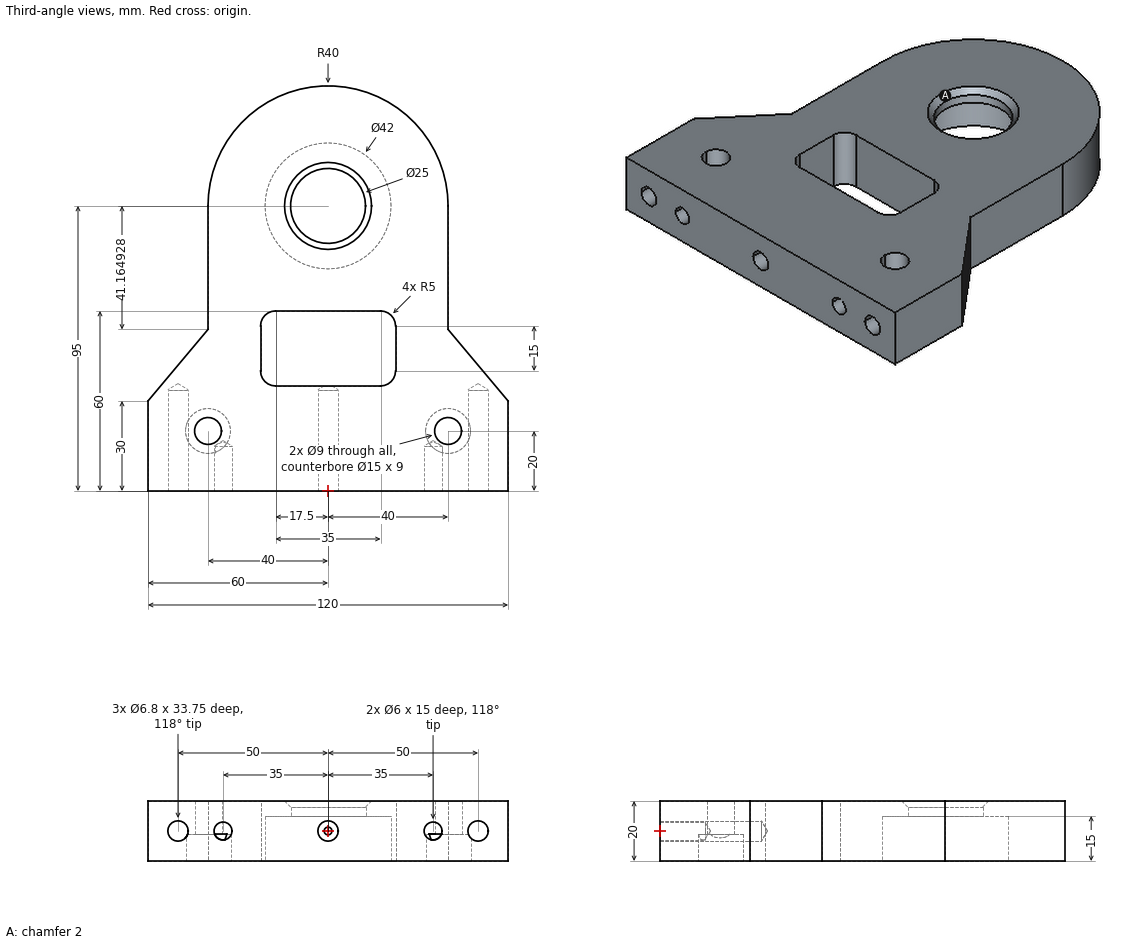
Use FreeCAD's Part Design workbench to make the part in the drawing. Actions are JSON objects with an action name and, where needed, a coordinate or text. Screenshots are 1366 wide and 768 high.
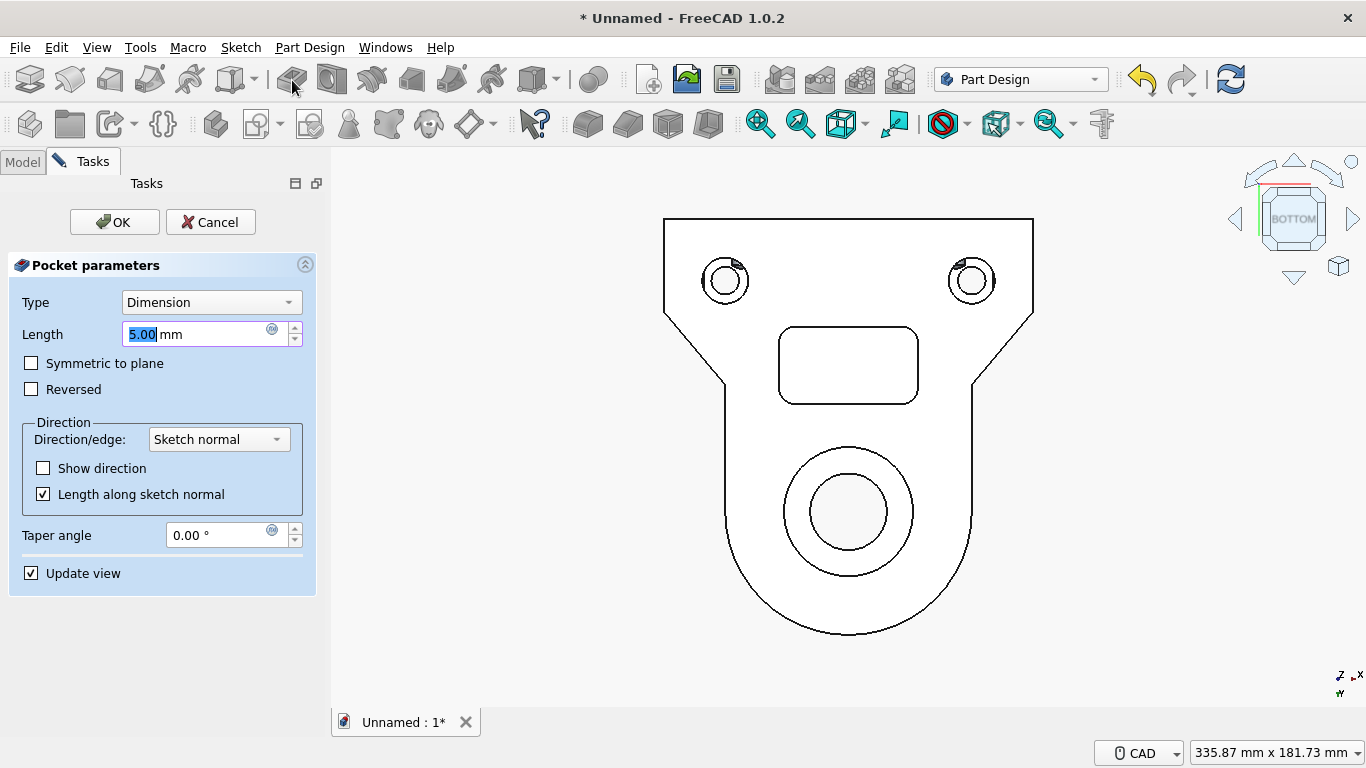
{"action": "left_click", "coordinate": [212, 302]}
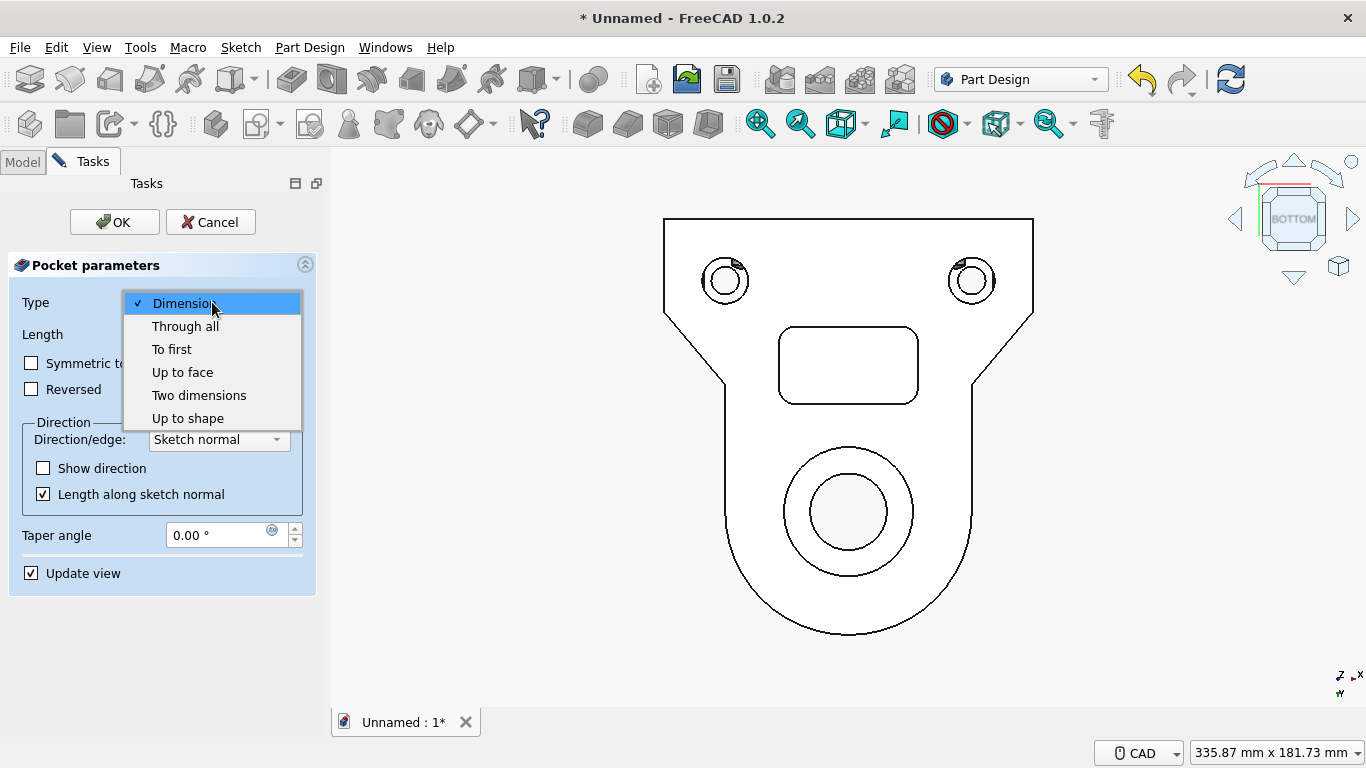
{"action": "left_click", "coordinate": [212, 326]}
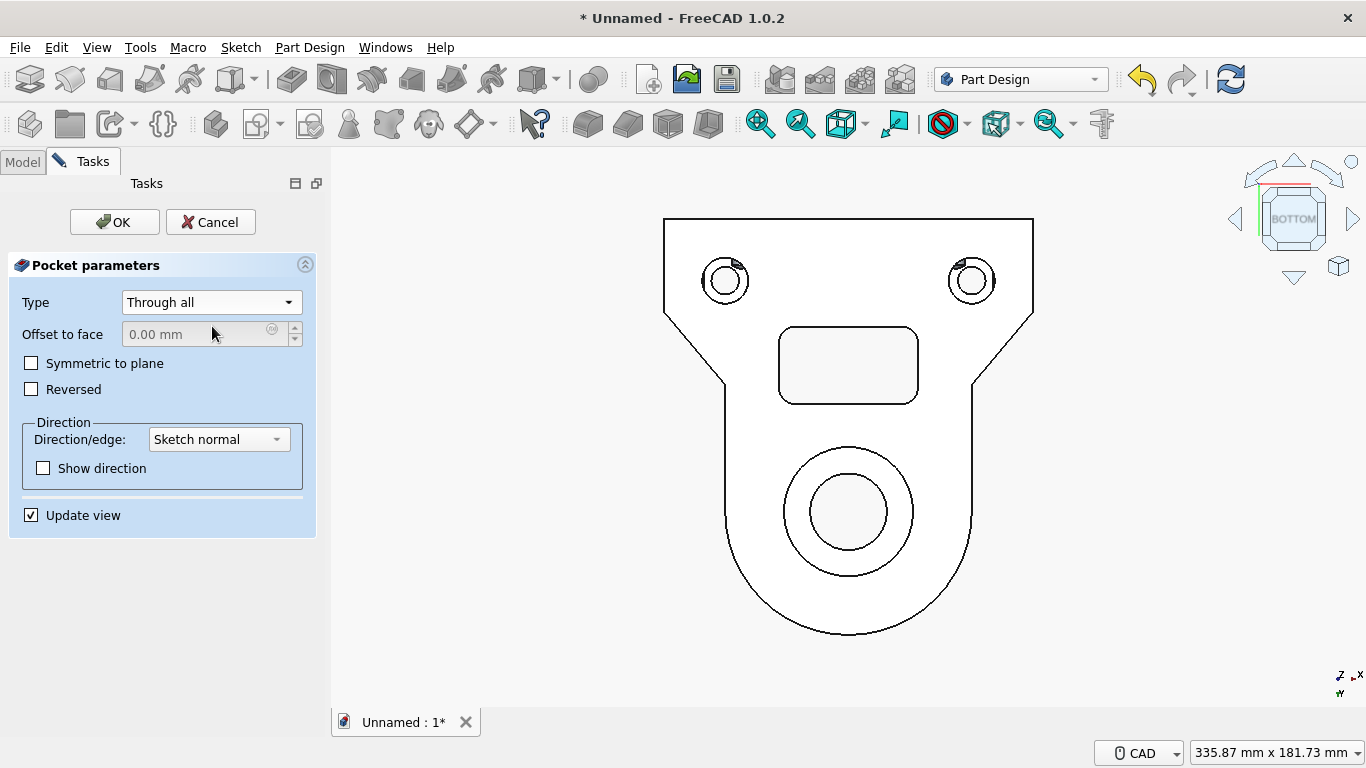
{"action": "left_click", "coordinate": [115, 222]}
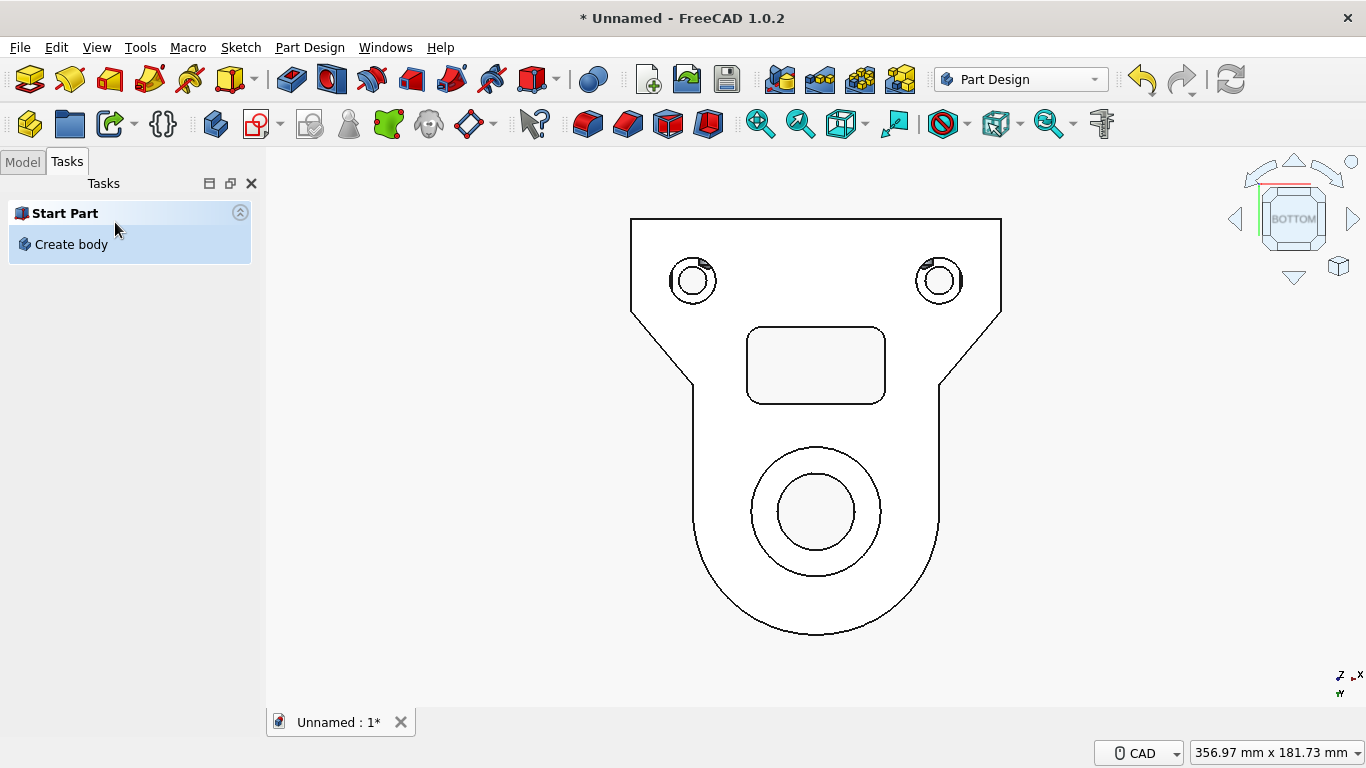
{"action": "key", "text": "0"}